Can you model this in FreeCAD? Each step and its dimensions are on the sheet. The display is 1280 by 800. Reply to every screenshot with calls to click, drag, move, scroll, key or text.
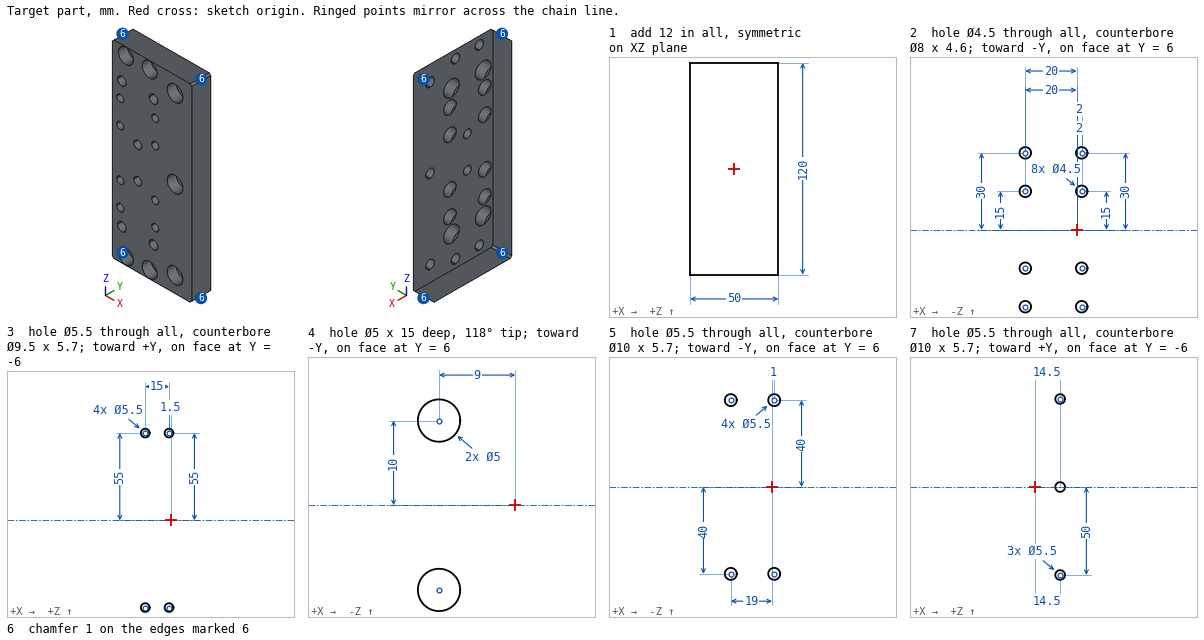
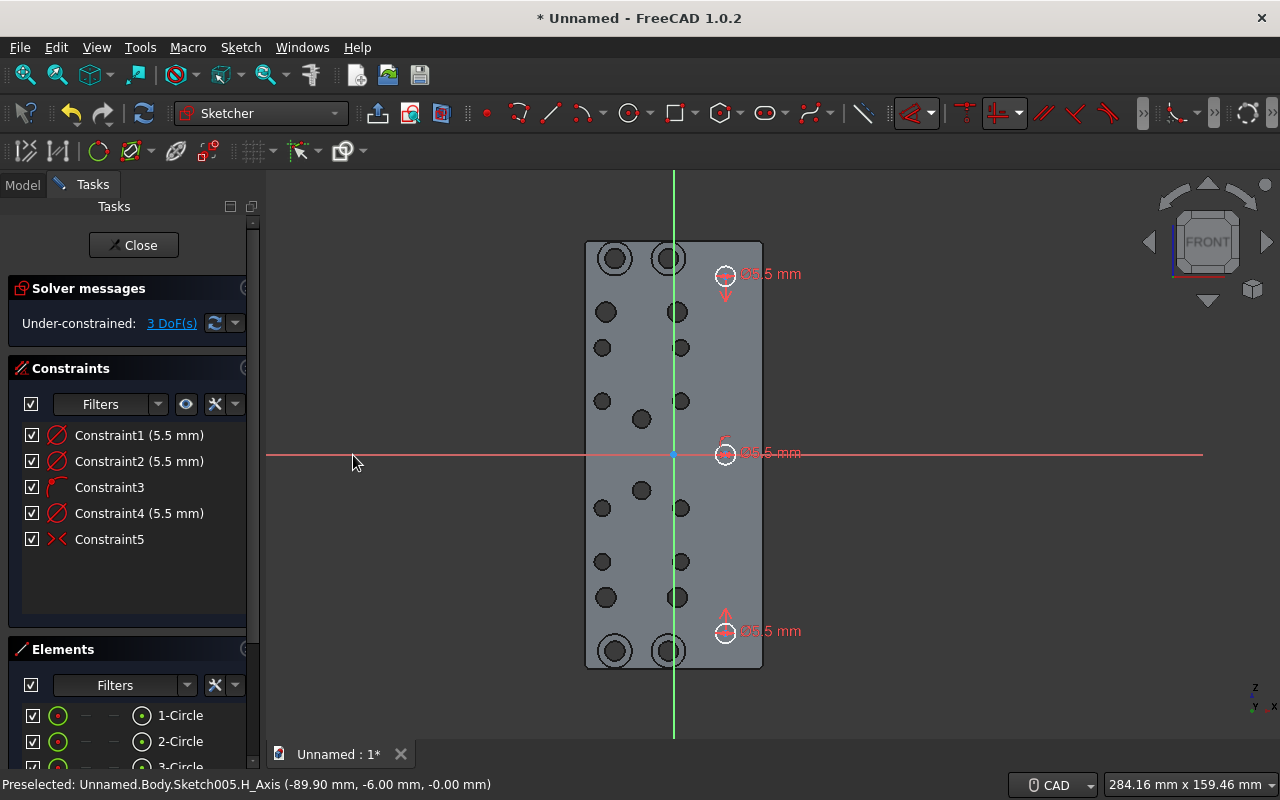
click(726, 633)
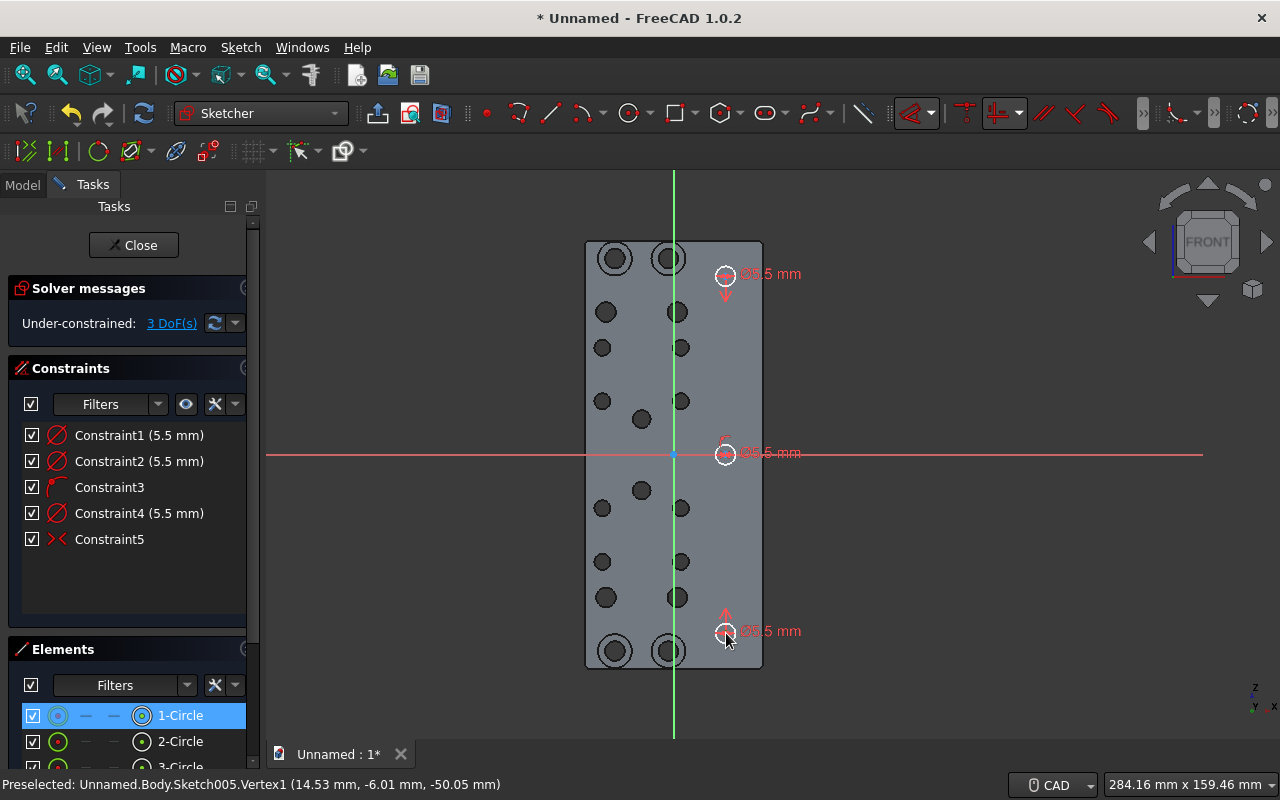
click(934, 114)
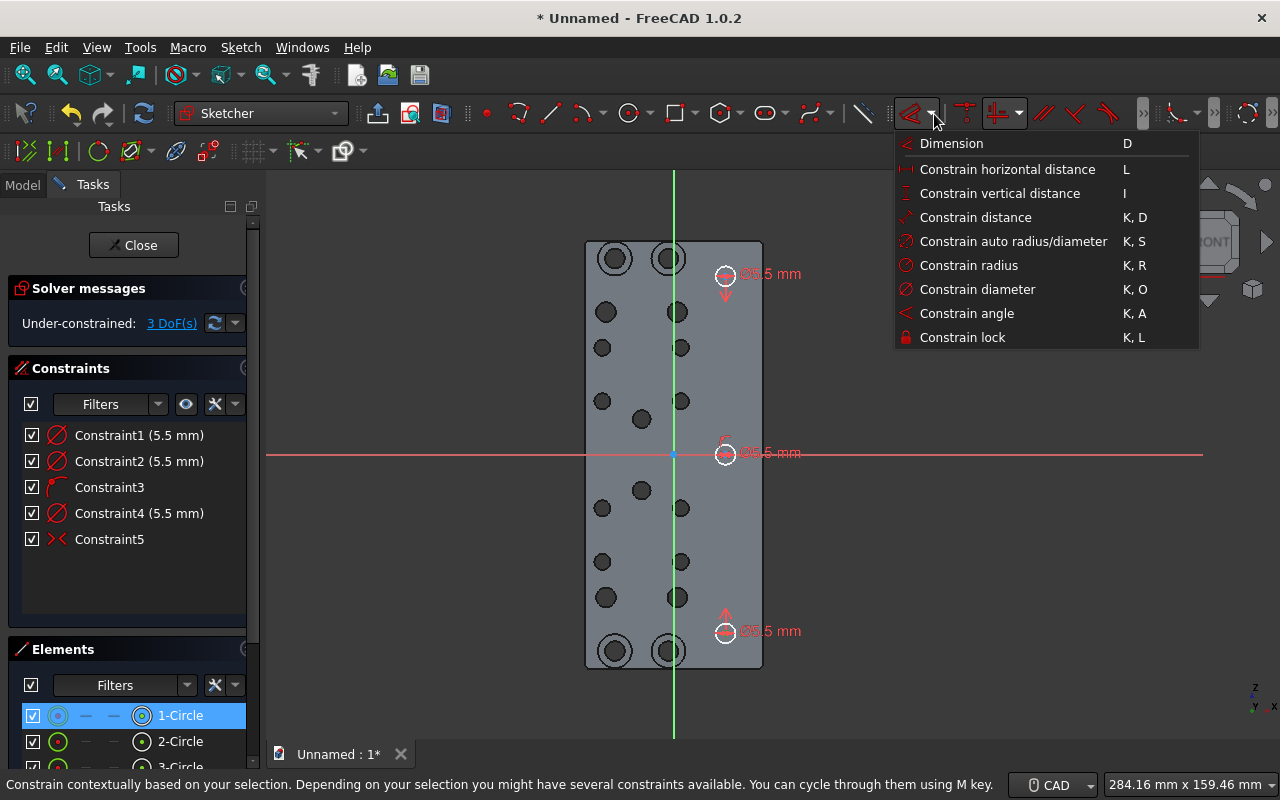
click(1047, 193)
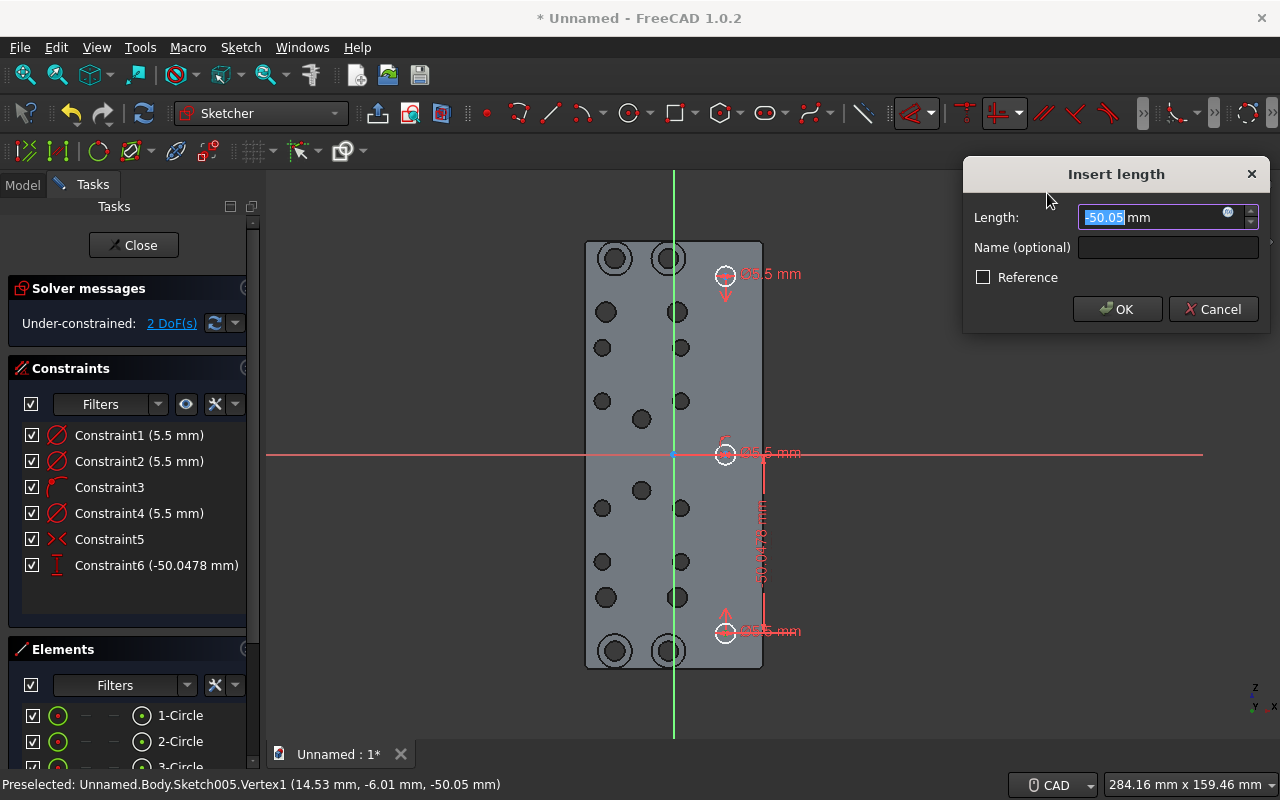
text(-50)
key(Return)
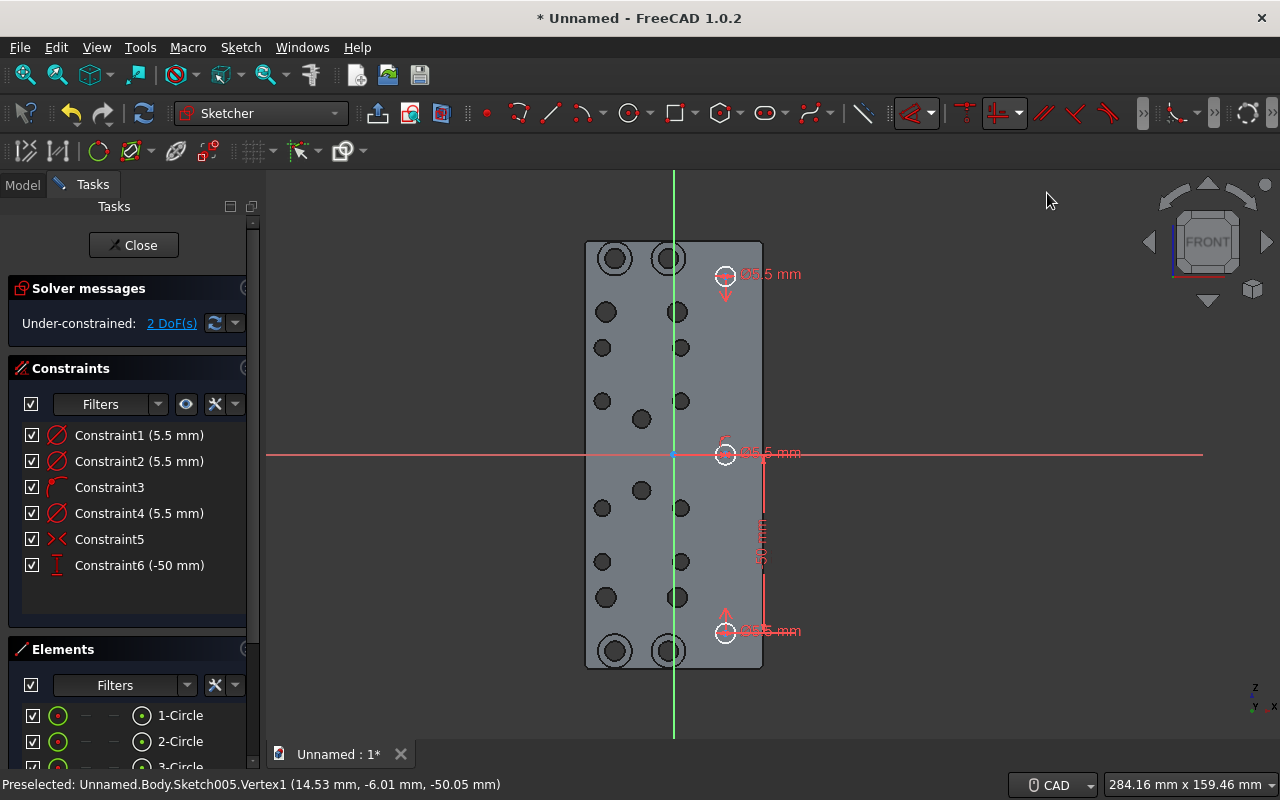
click(726, 633)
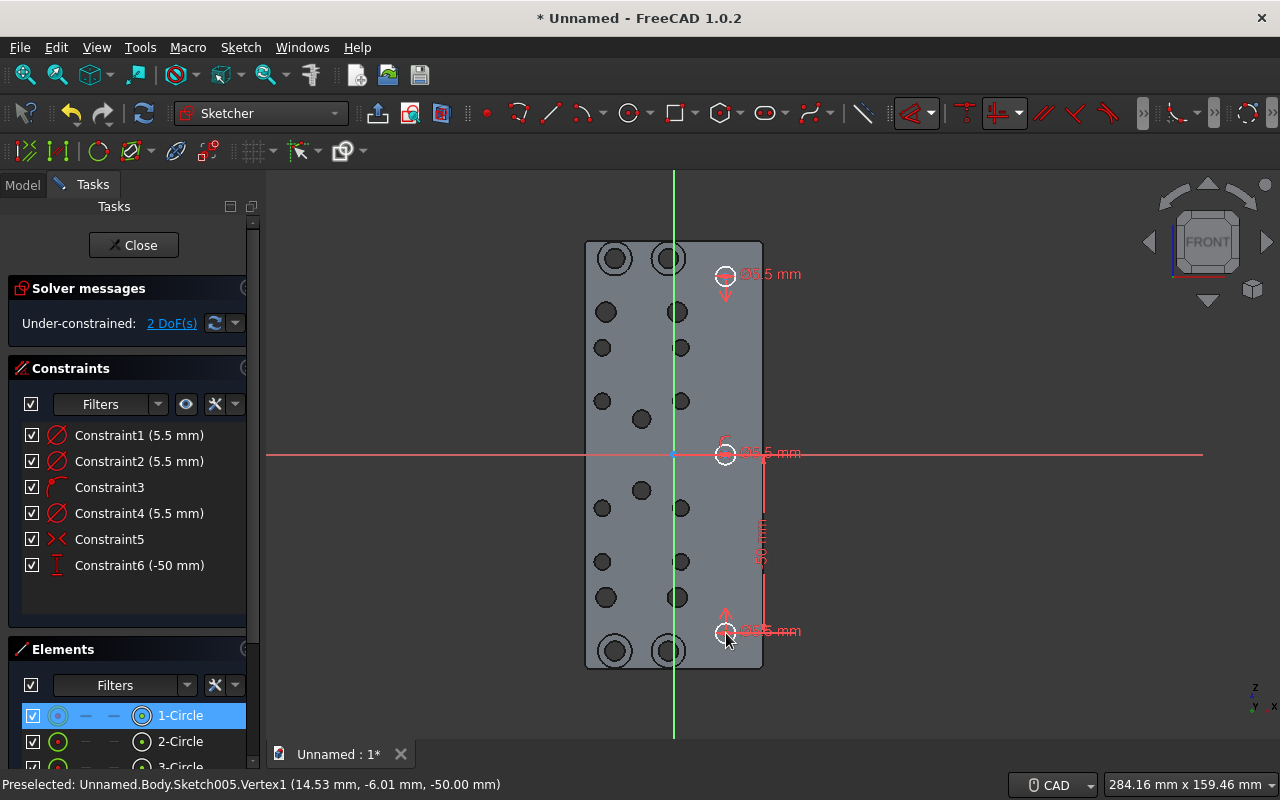
key(l)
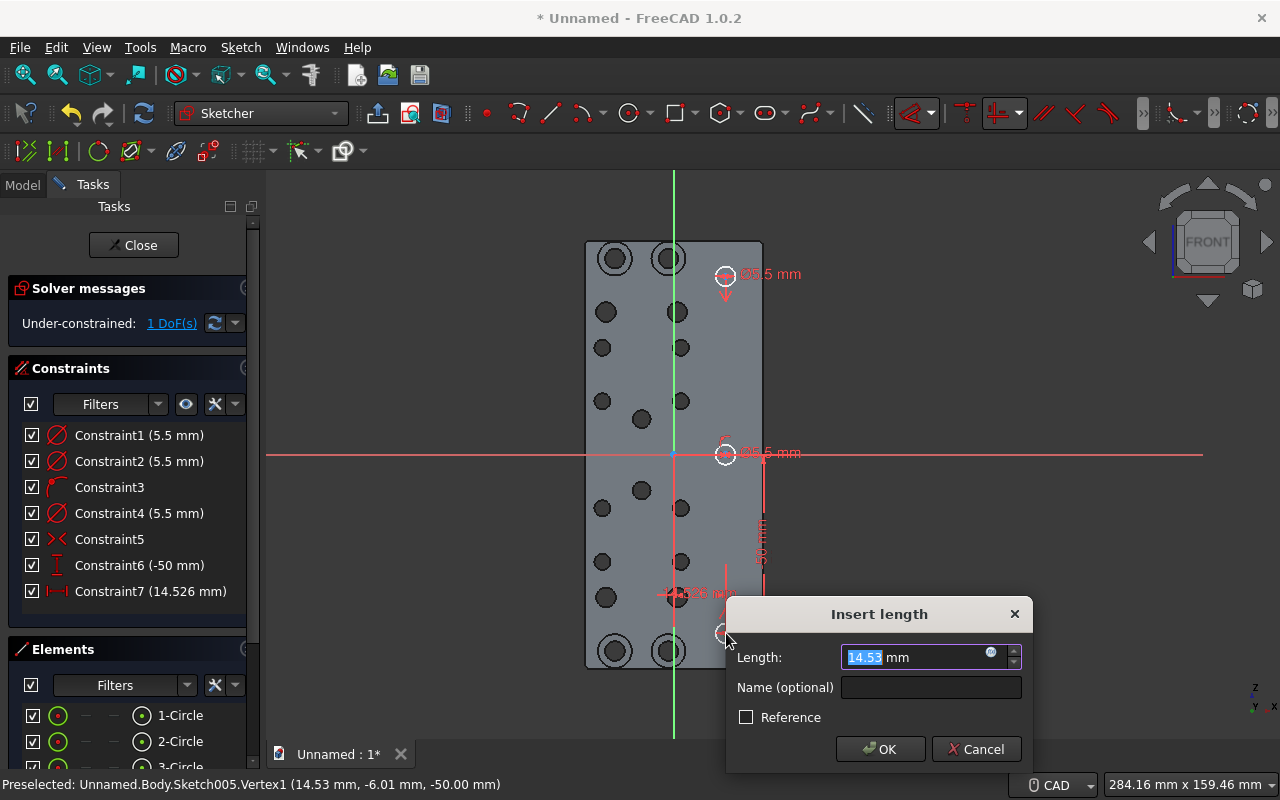
text(14.5)
key(Return)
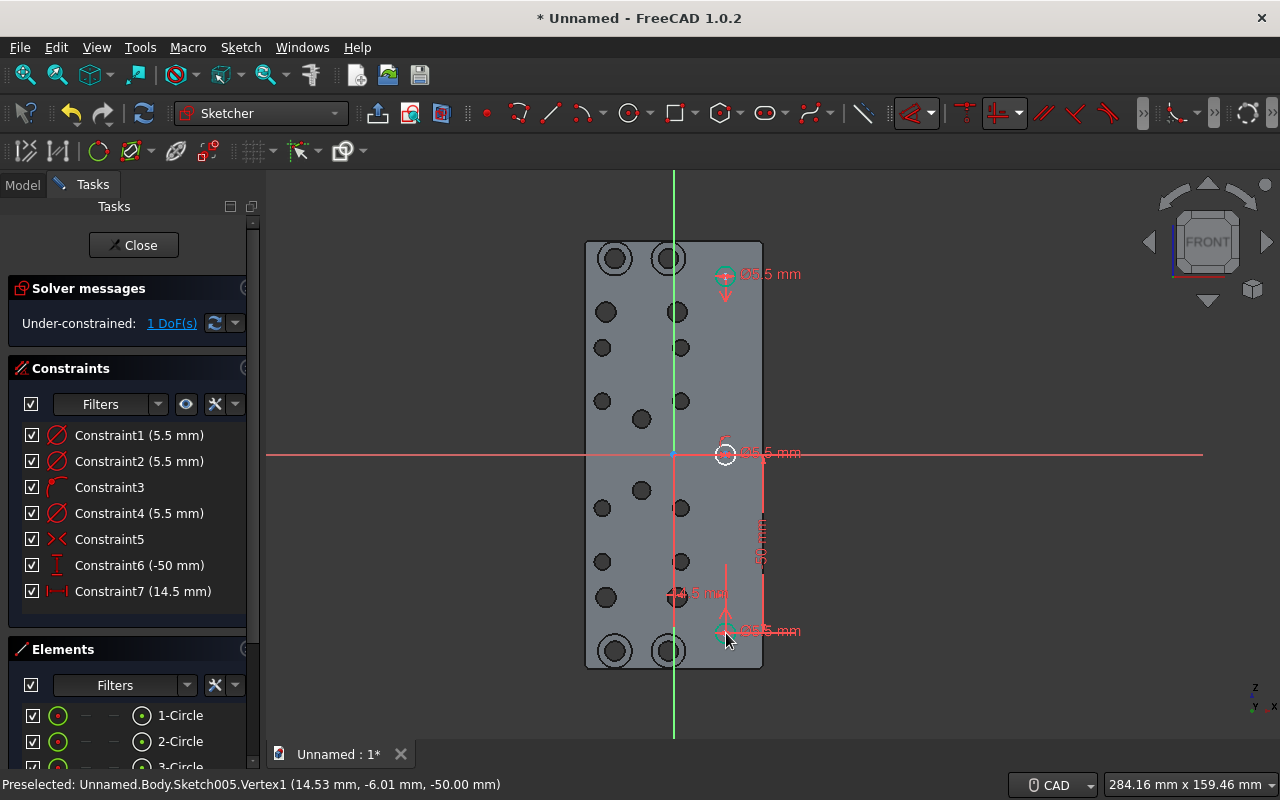
click(726, 455)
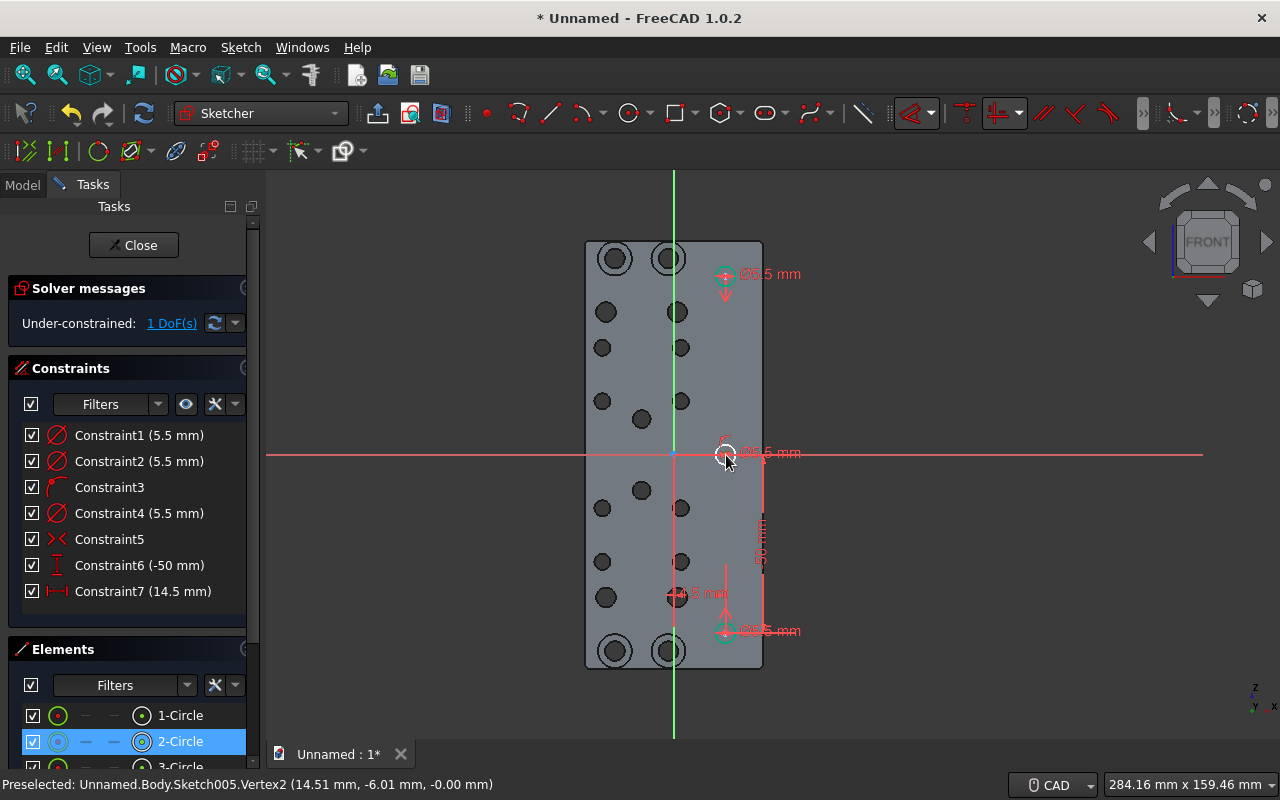
click(934, 114)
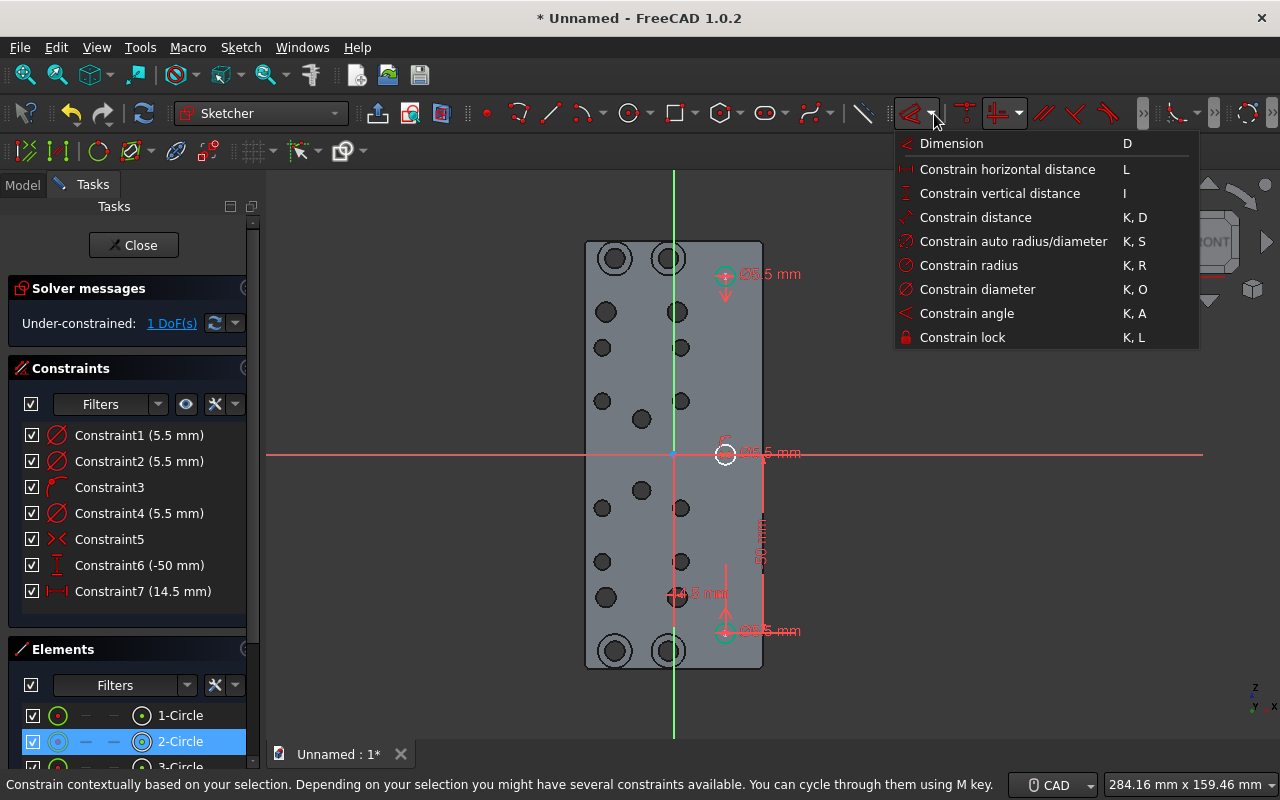
click(1047, 169)